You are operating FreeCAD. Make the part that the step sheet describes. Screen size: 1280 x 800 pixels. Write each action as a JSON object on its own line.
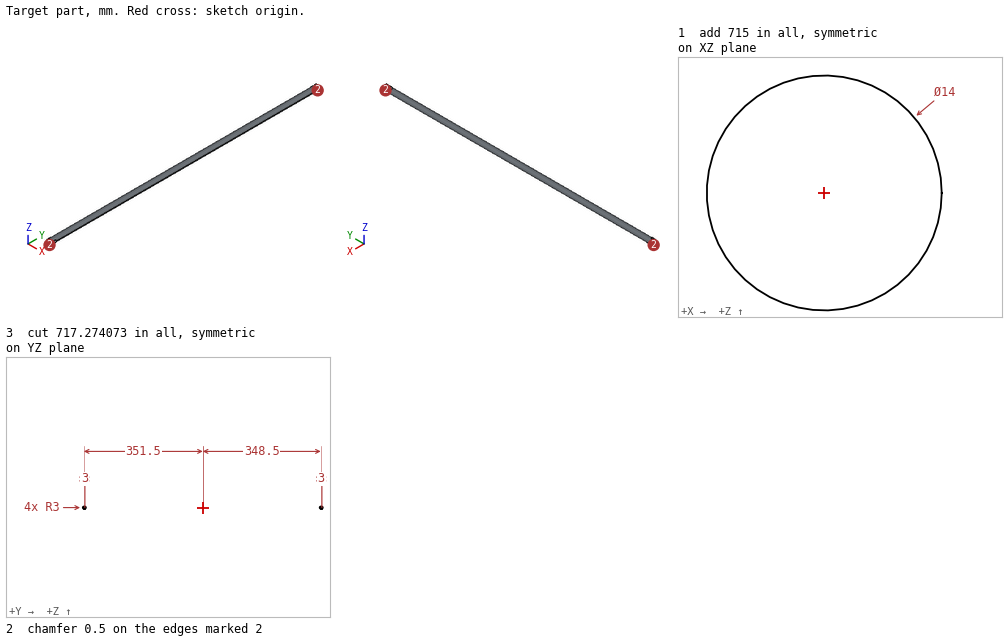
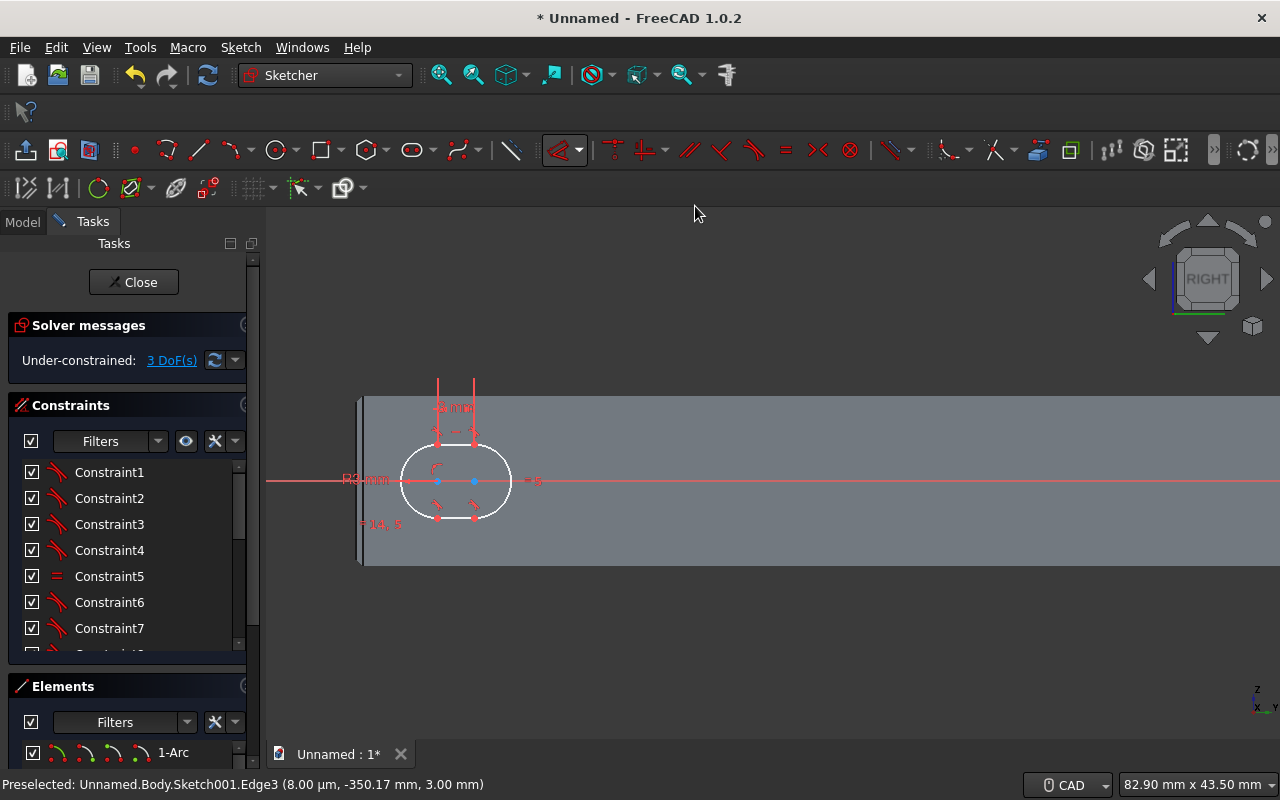
{"action": "scroll", "coordinate": [444, 472], "scroll_direction": "down", "scroll_amount": 14}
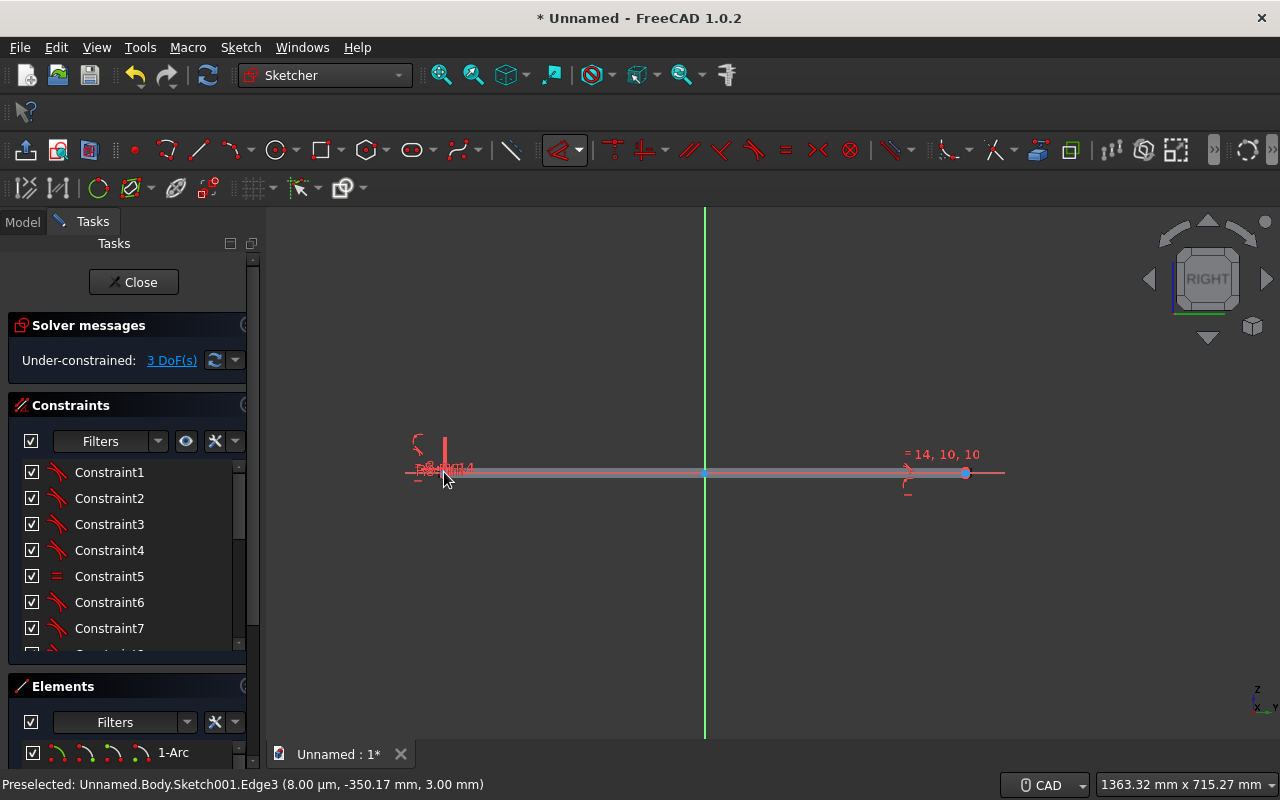
{"action": "scroll", "coordinate": [965, 471], "scroll_direction": "up", "scroll_amount": 15}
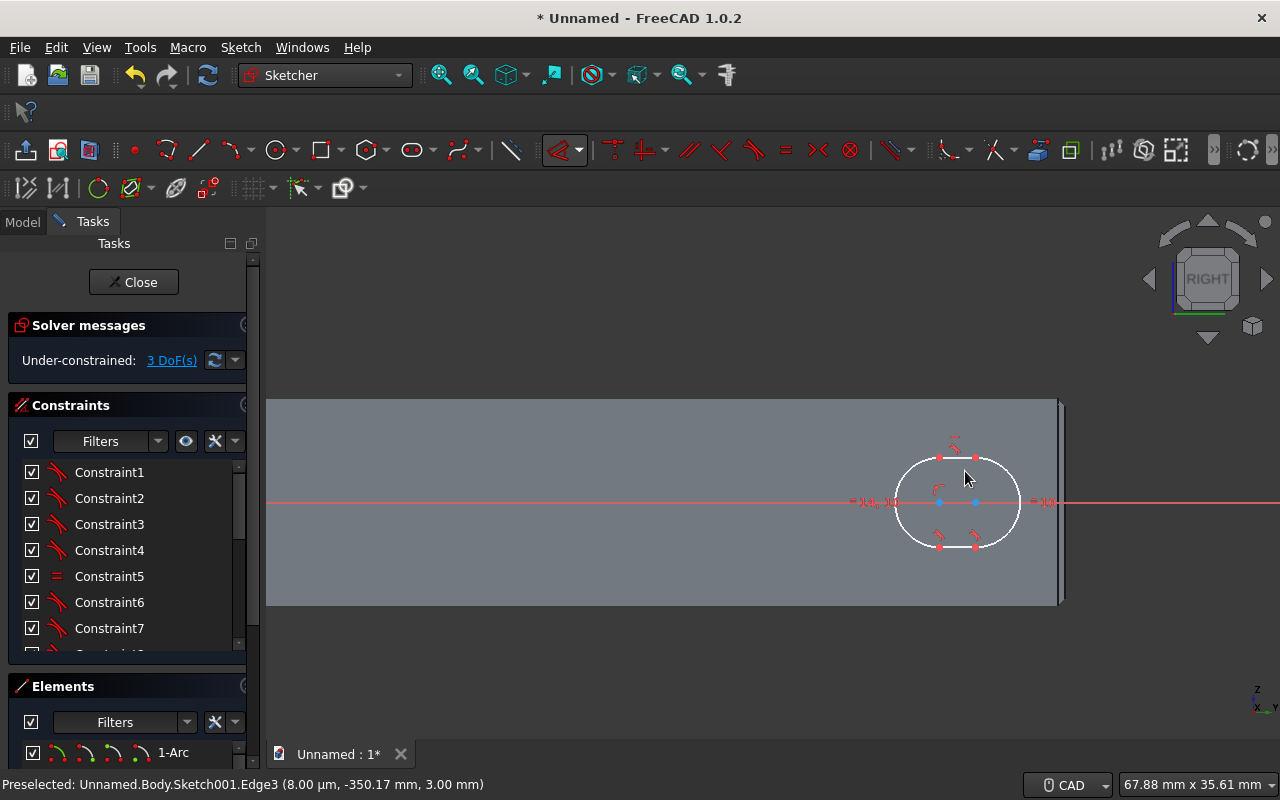
{"action": "left_click", "coordinate": [954, 458]}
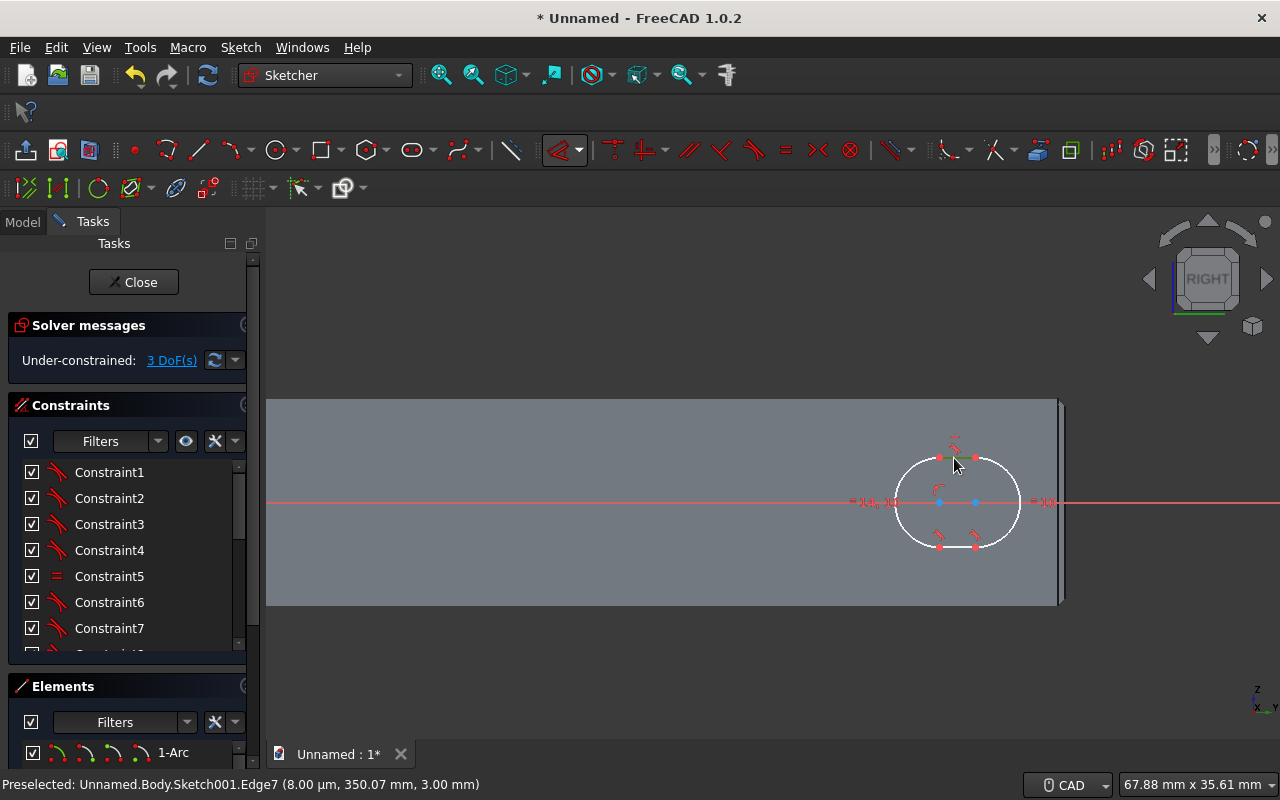
{"action": "left_click", "coordinate": [582, 150]}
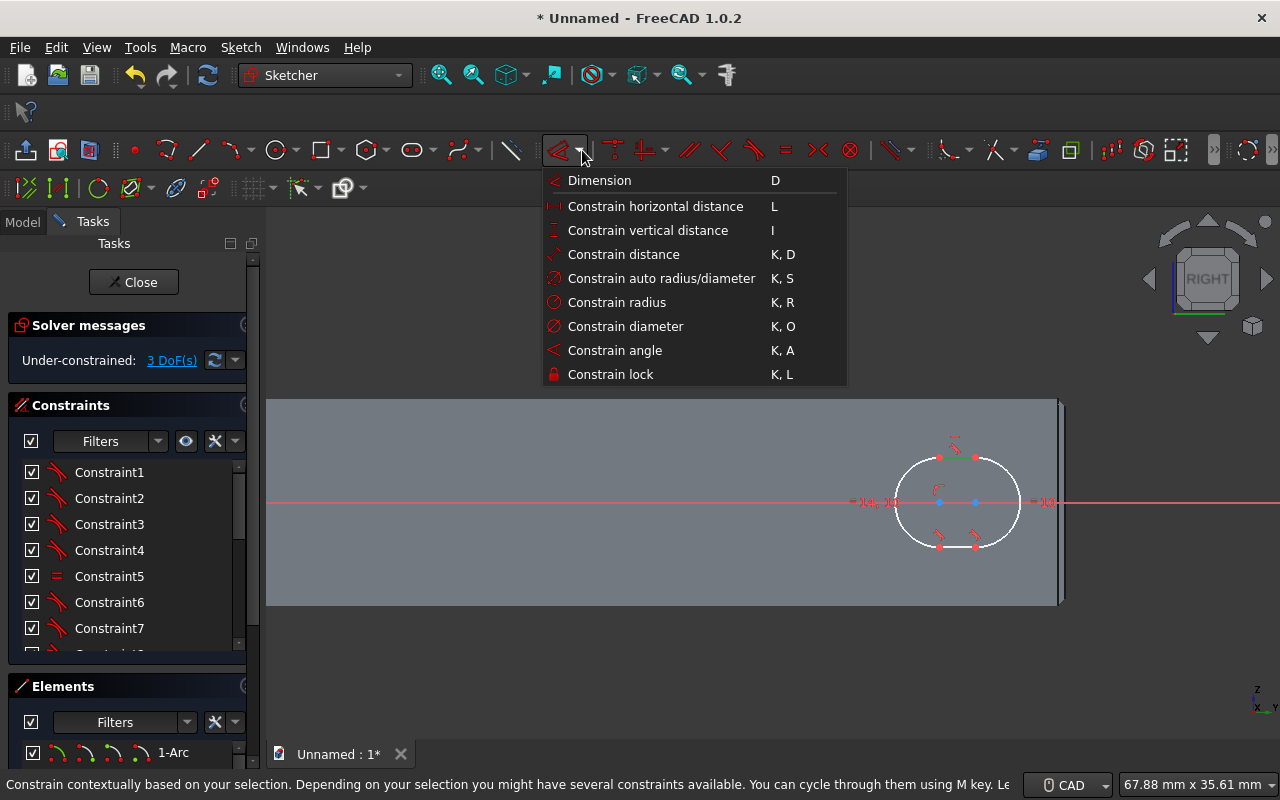
{"action": "left_click", "coordinate": [695, 206]}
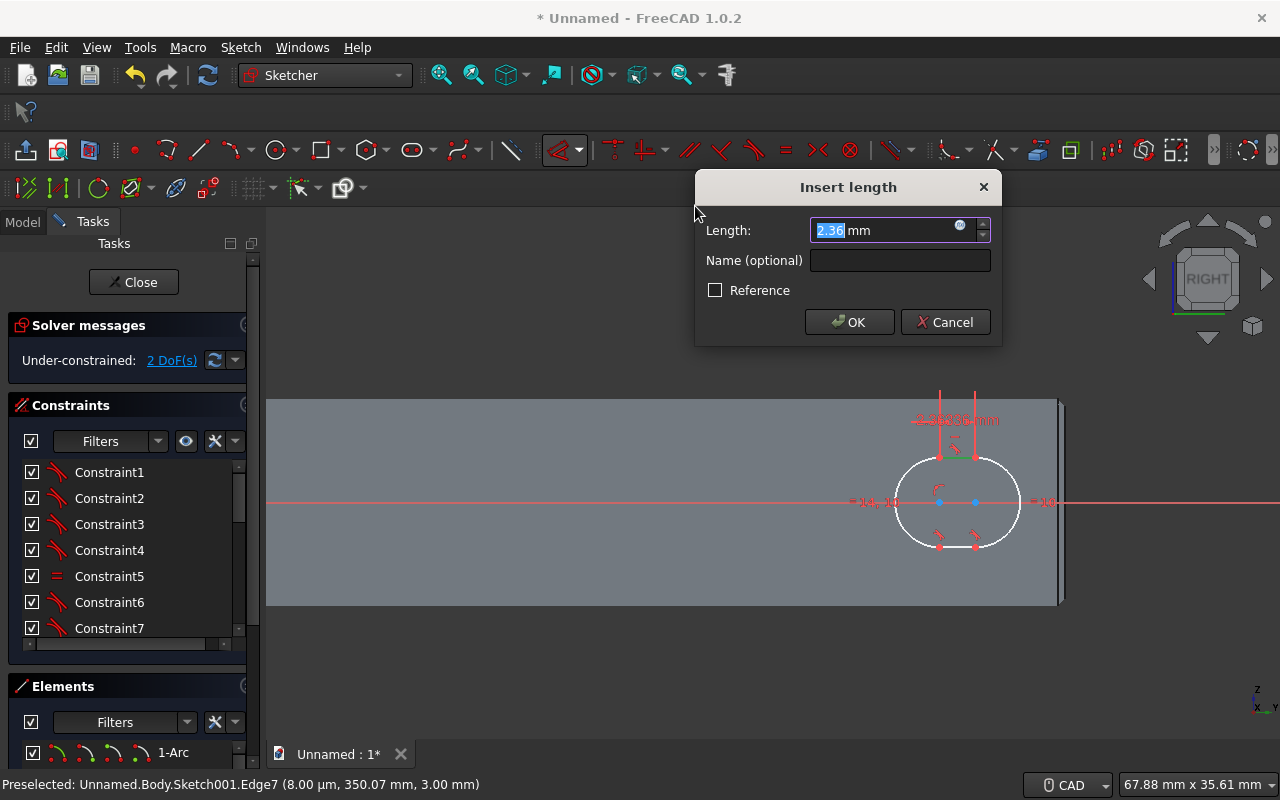
{"action": "type", "text": "3"}
{"action": "key", "text": "Return"}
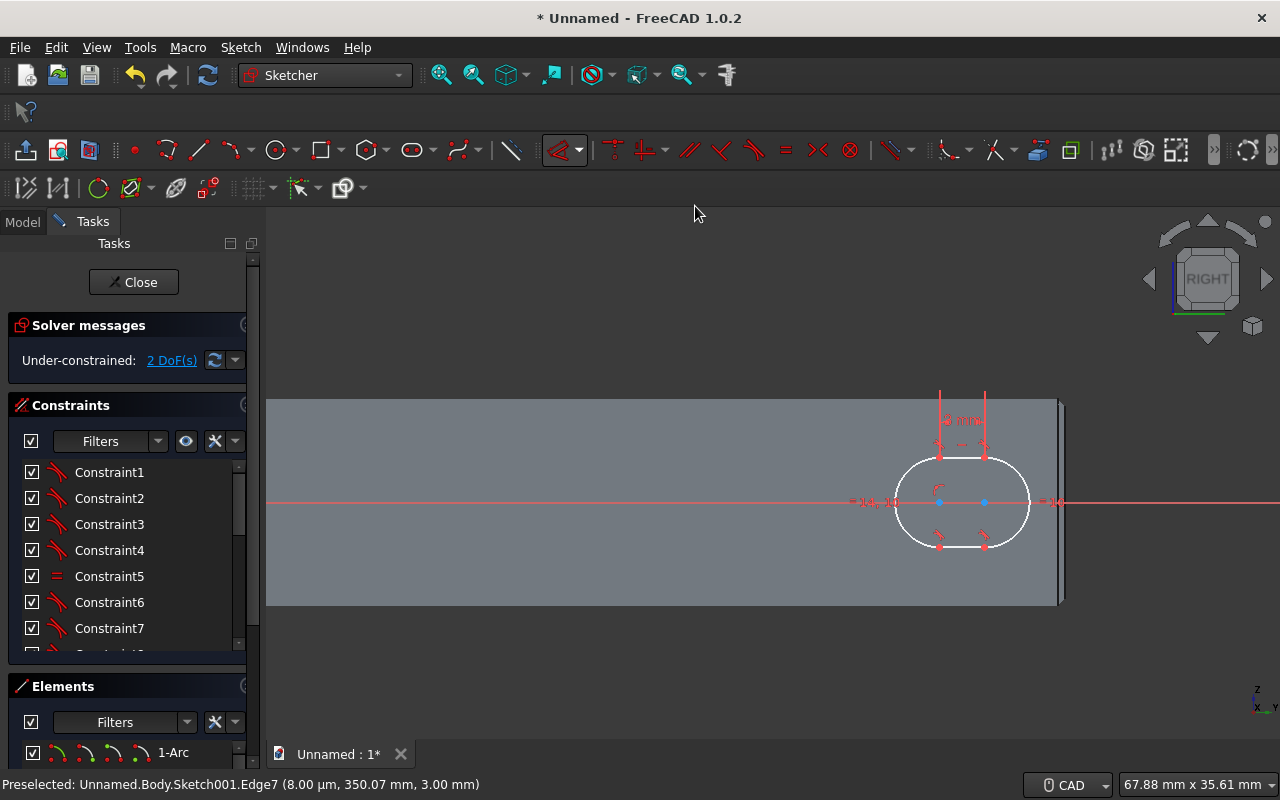
{"action": "scroll", "coordinate": [965, 471], "scroll_direction": "down", "scroll_amount": 15}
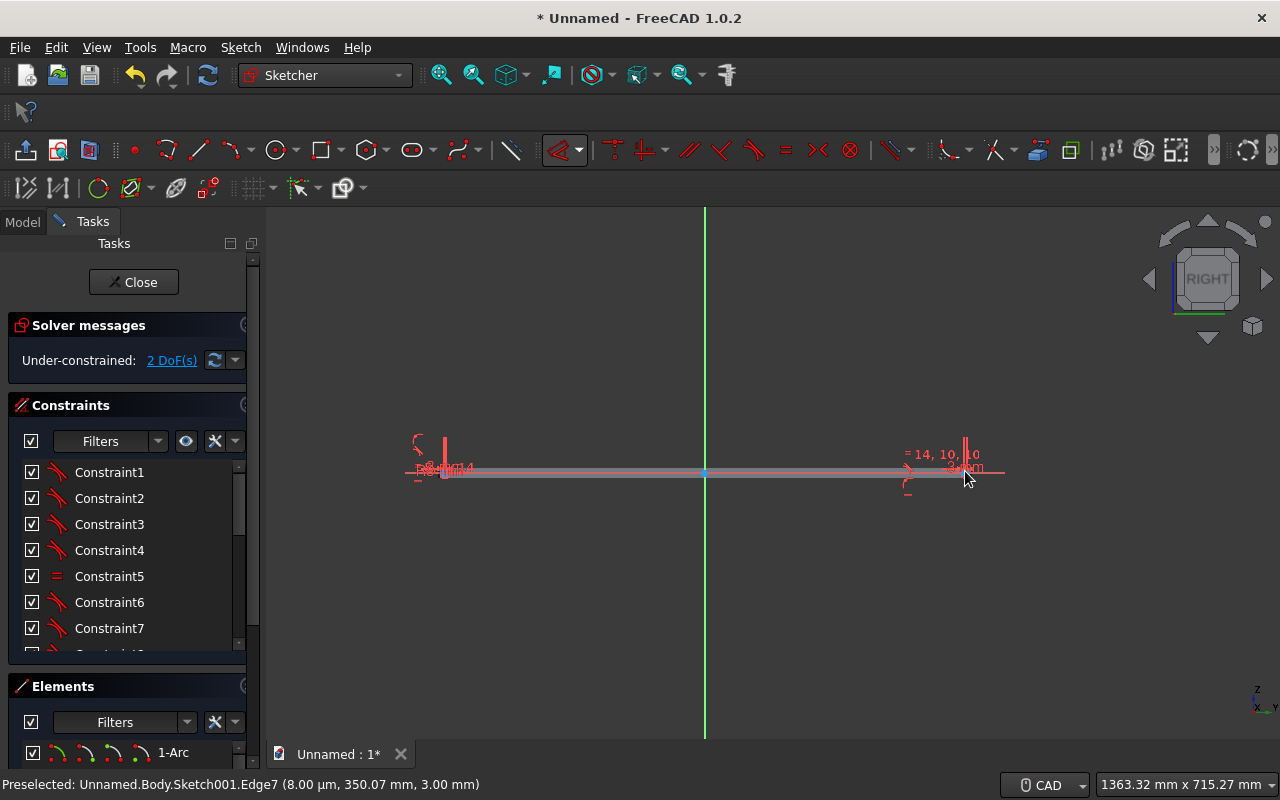
{"action": "scroll", "coordinate": [444, 471], "scroll_direction": "up", "scroll_amount": 9}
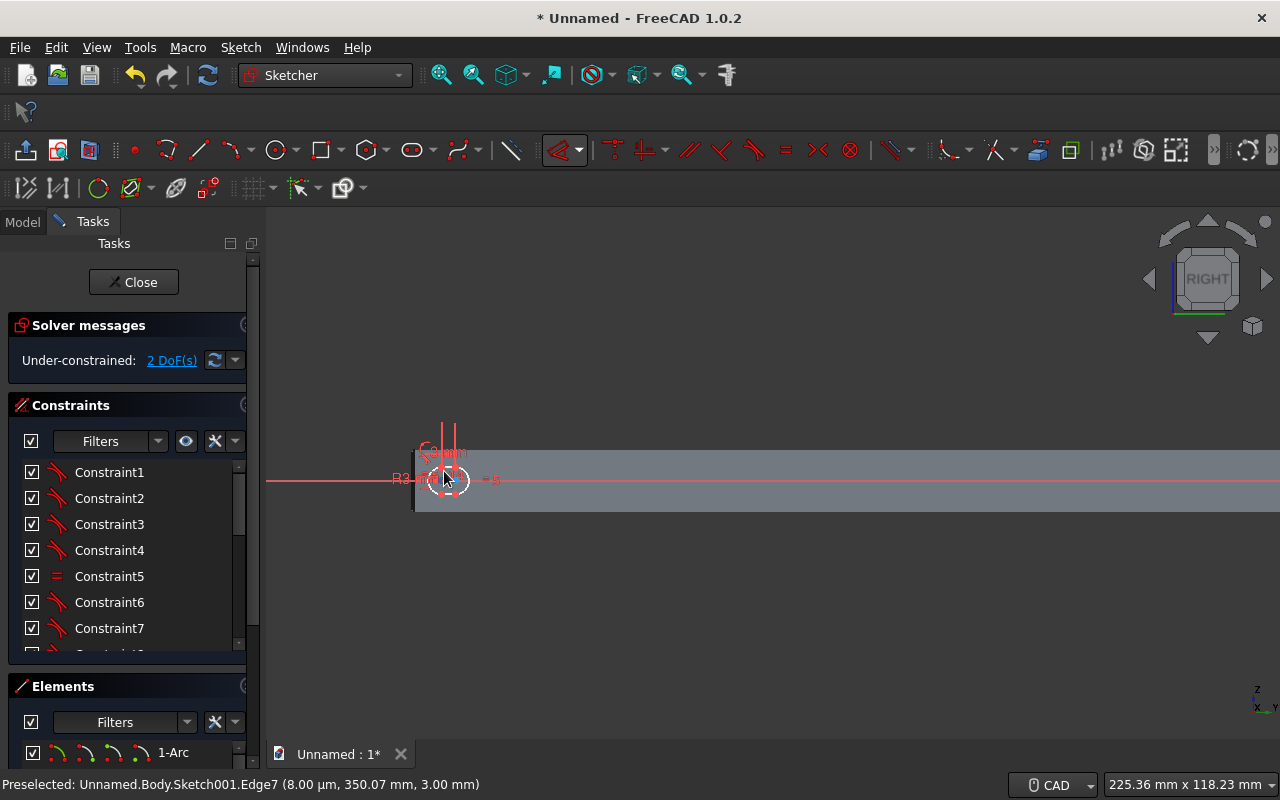
{"action": "left_click", "coordinate": [442, 467]}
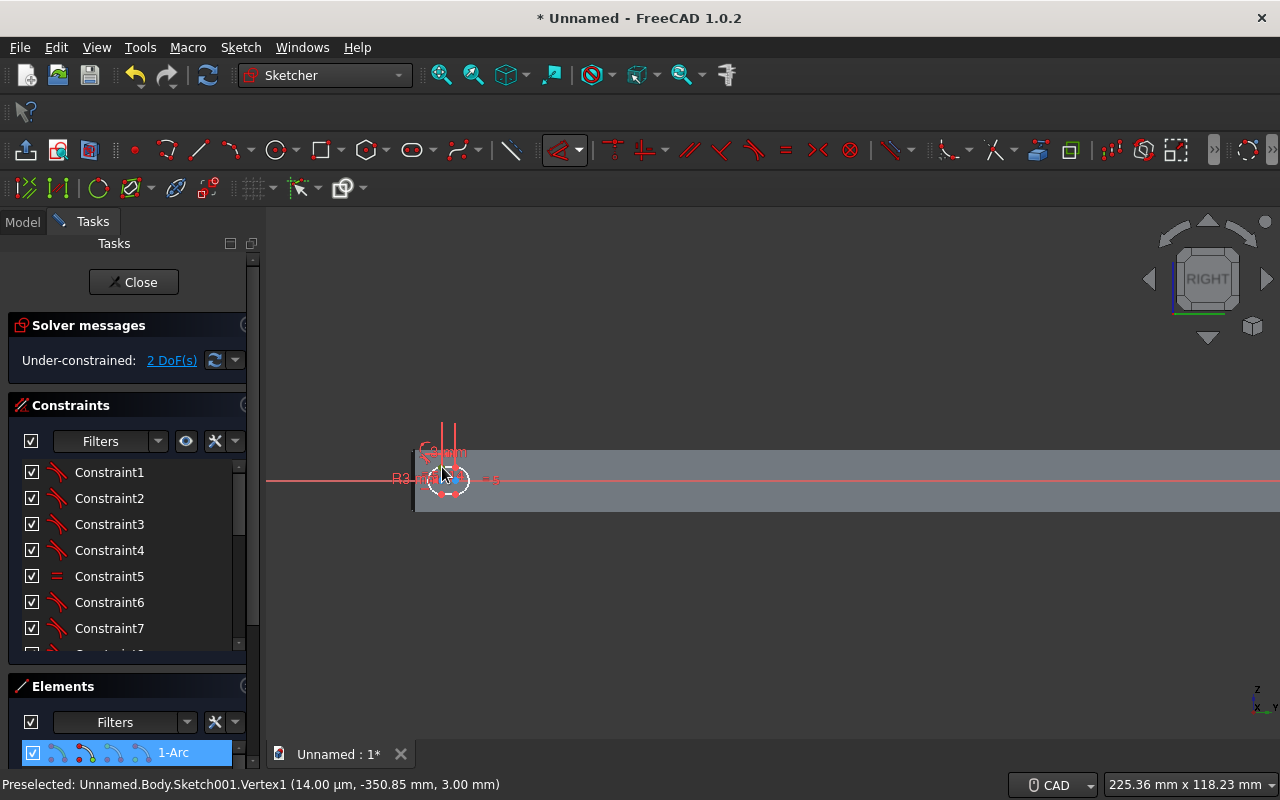
{"action": "key", "text": "l"}